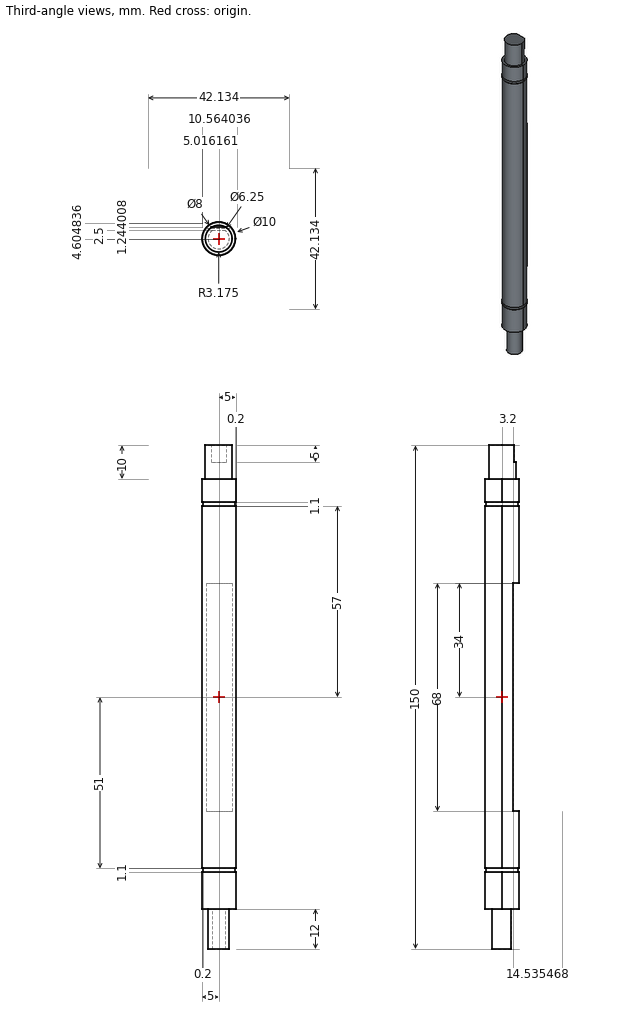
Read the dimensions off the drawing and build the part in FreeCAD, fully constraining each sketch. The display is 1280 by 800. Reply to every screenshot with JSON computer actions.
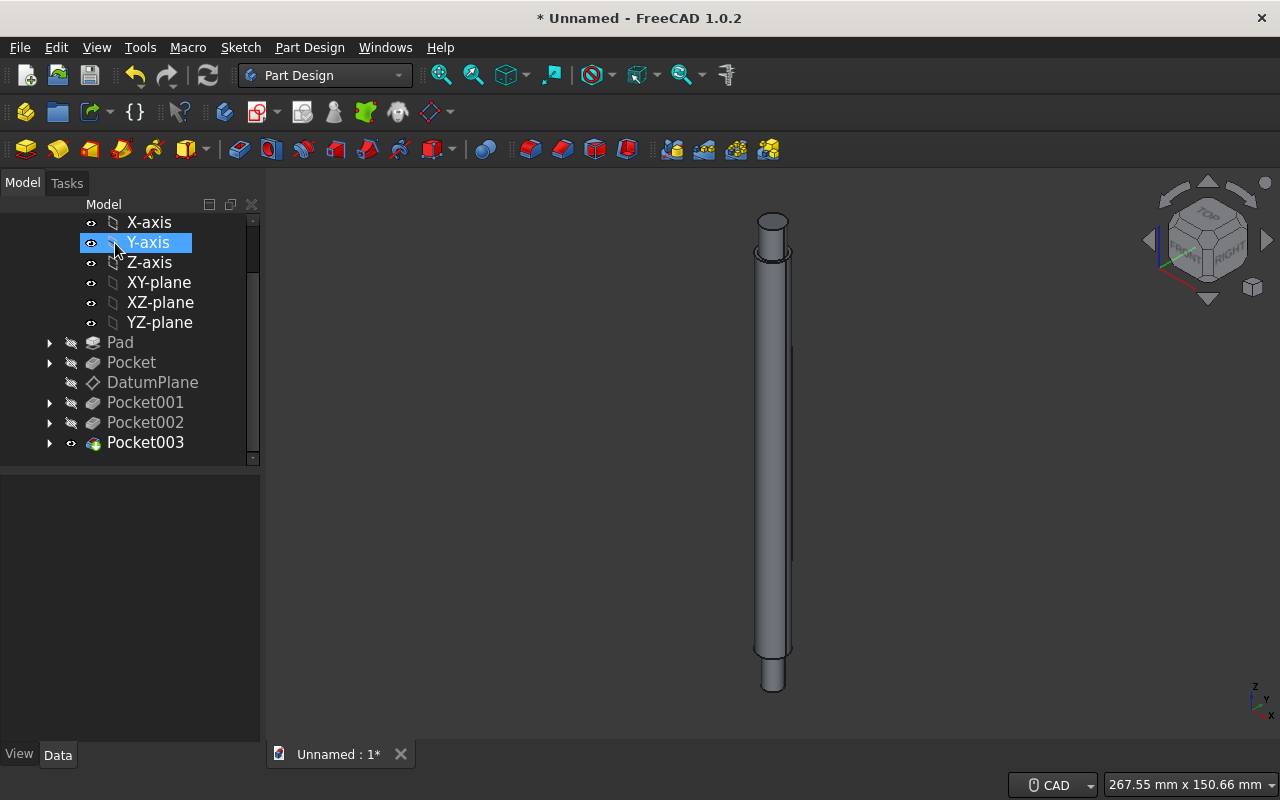
{"action": "left_click", "coordinate": [773, 220]}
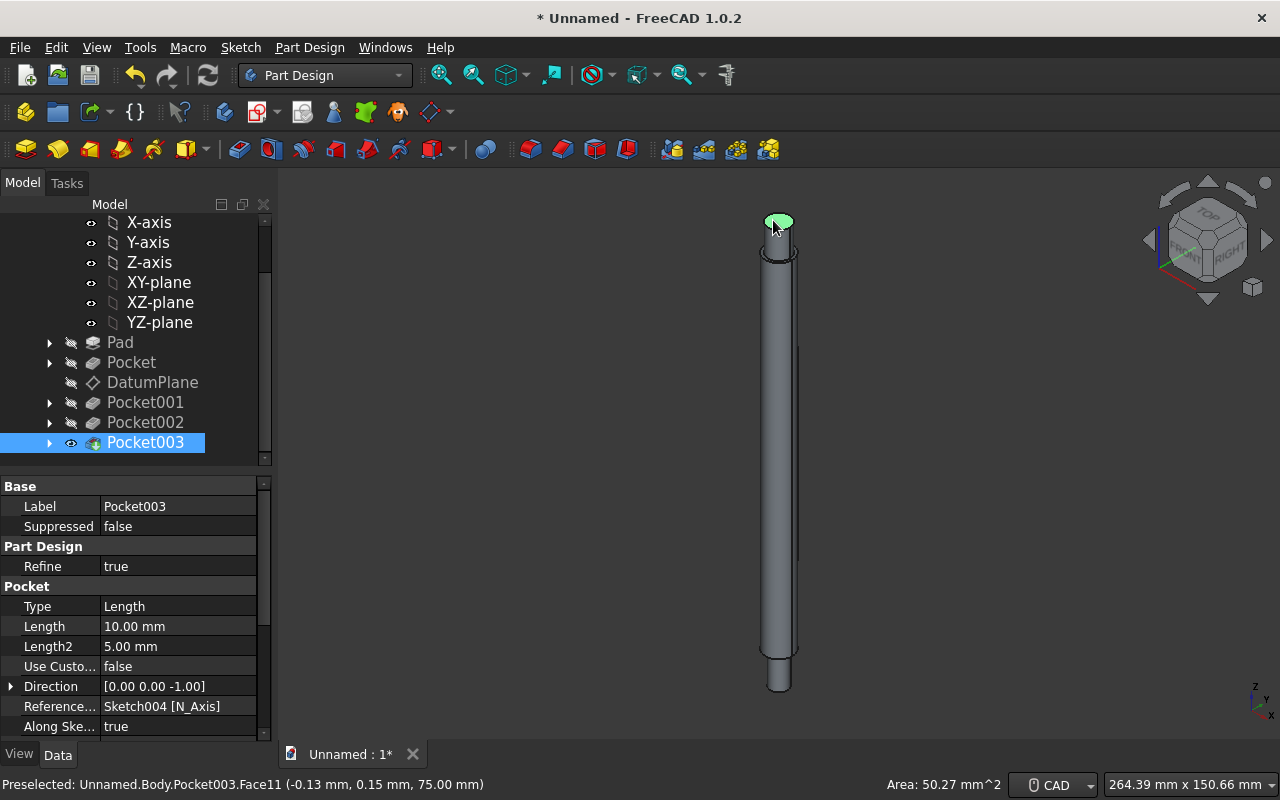
{"action": "left_click", "coordinate": [258, 112]}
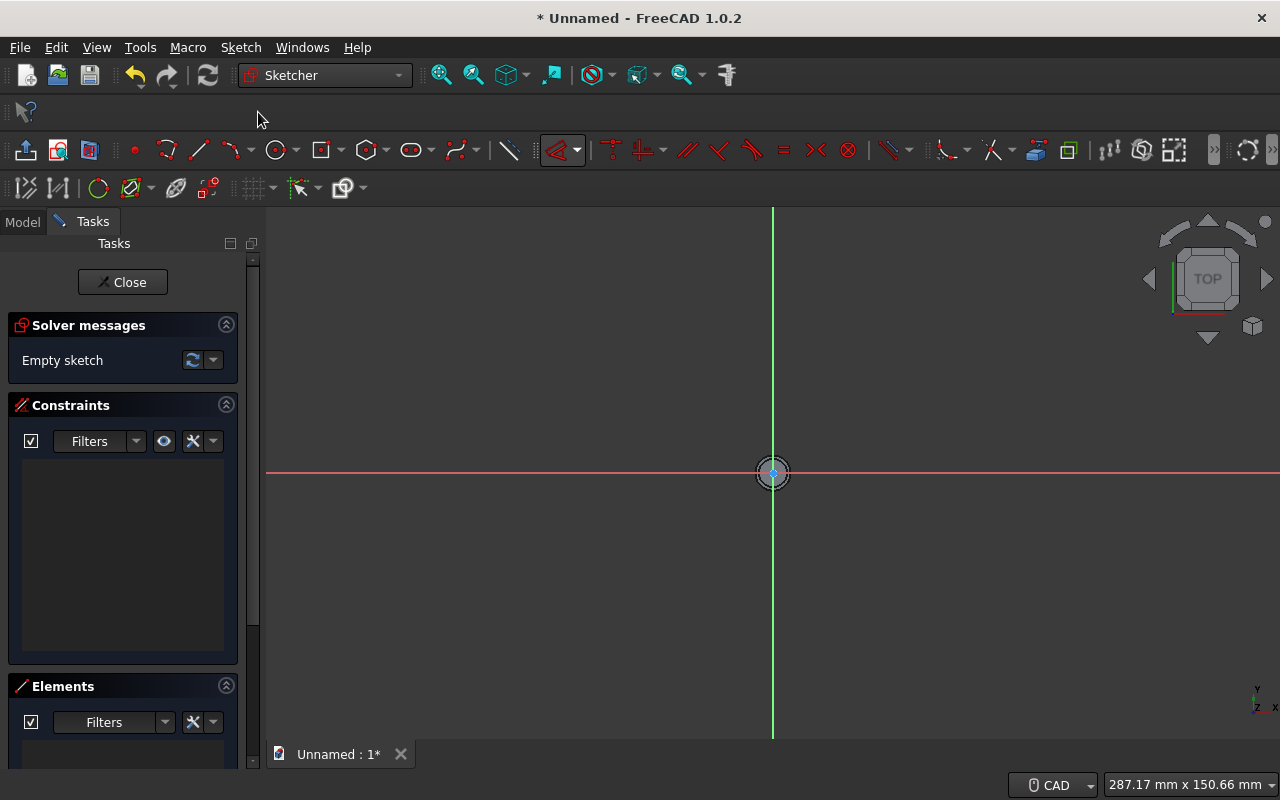
{"action": "scroll", "coordinate": [778, 464], "scroll_direction": "up", "scroll_amount": 14}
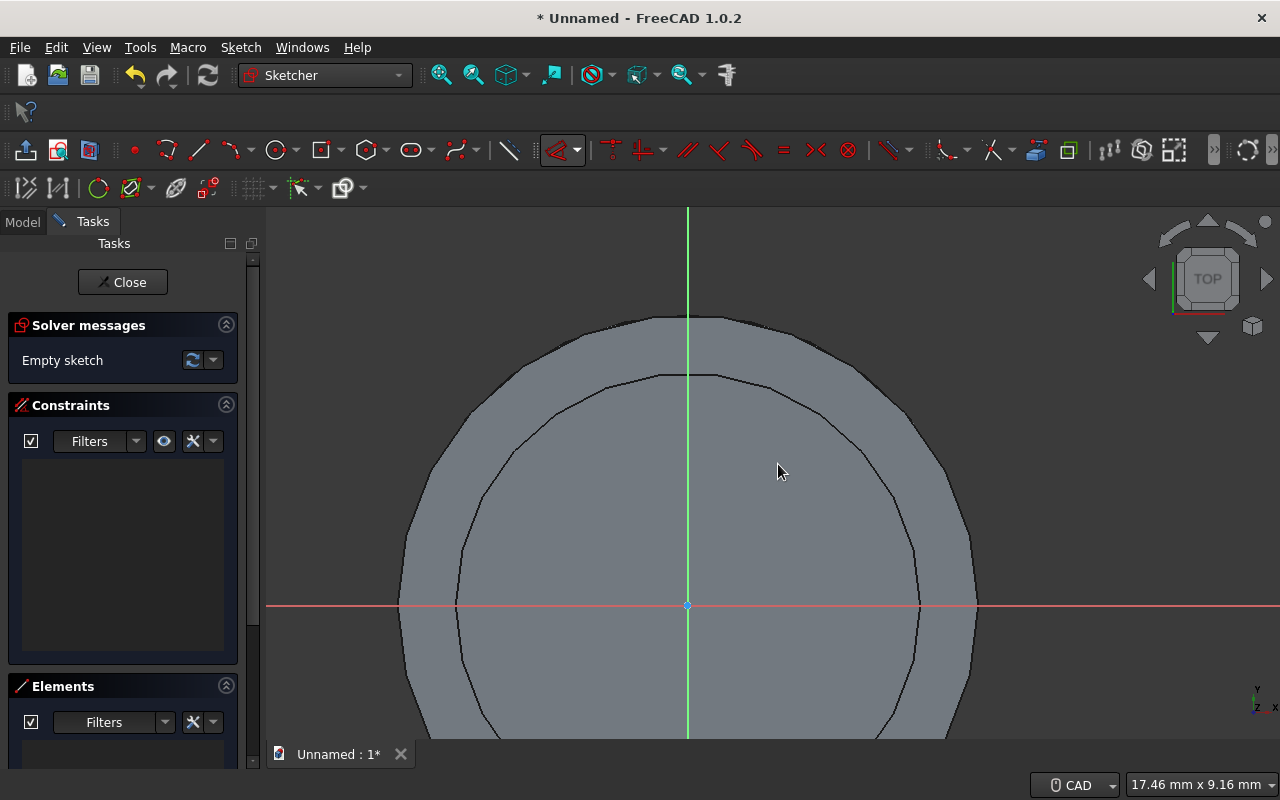
{"action": "key", "text": "g r"}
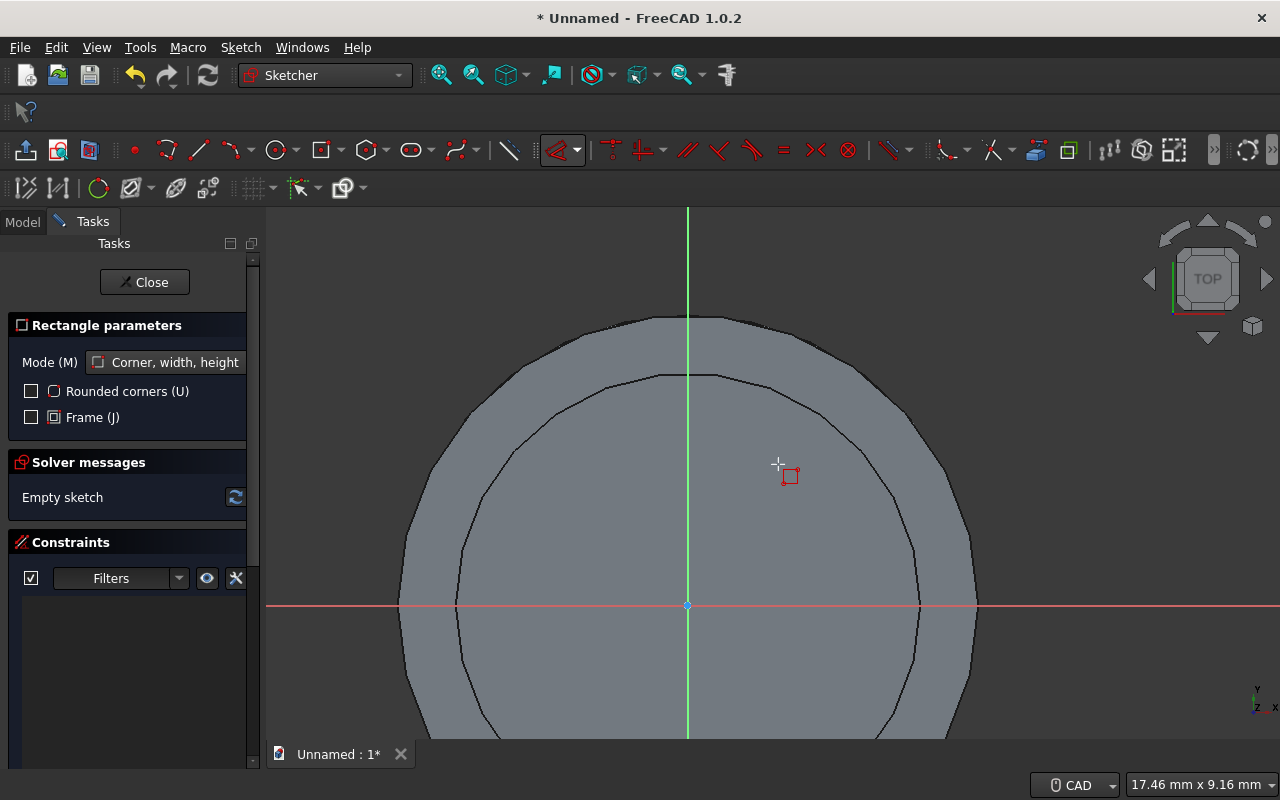
{"action": "left_click", "coordinate": [397, 338]}
{"action": "left_click", "coordinate": [1010, 410]}
{"action": "key", "text": "Escape"}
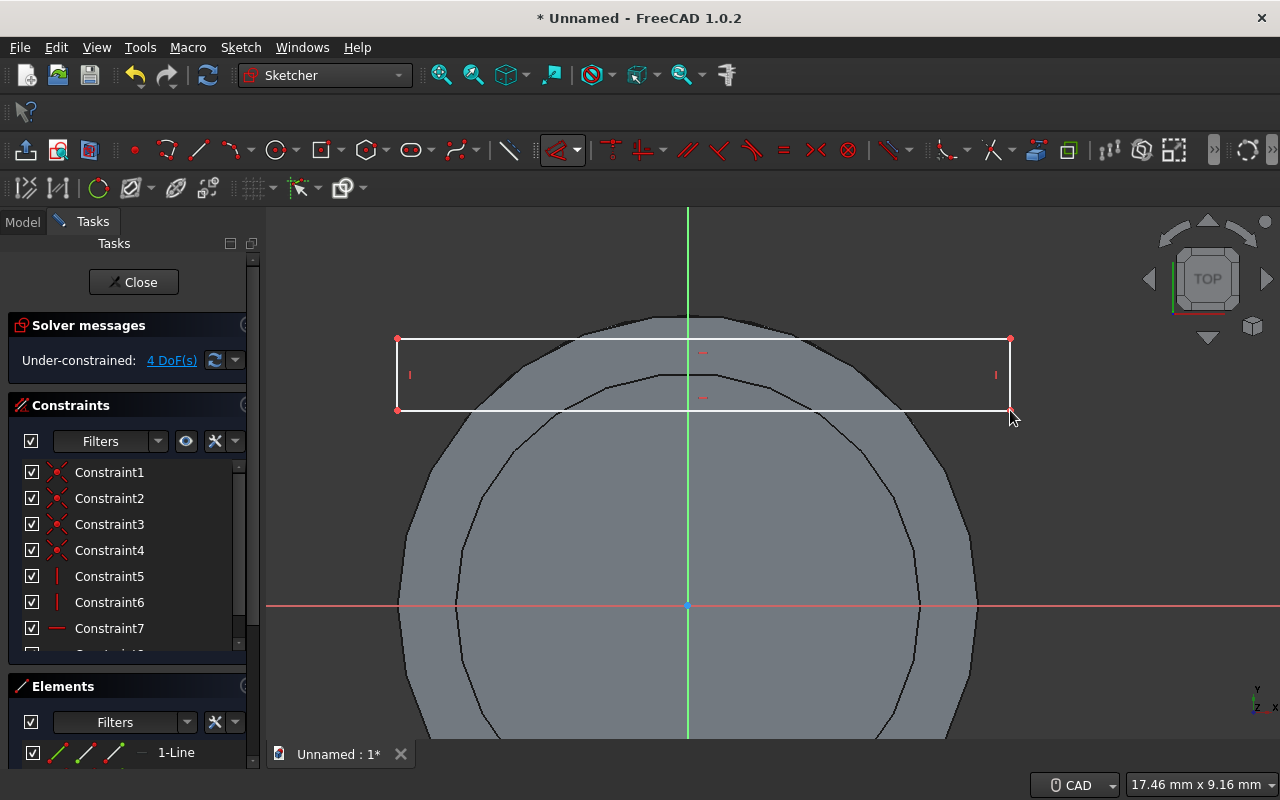
{"action": "left_click", "coordinate": [397, 361]}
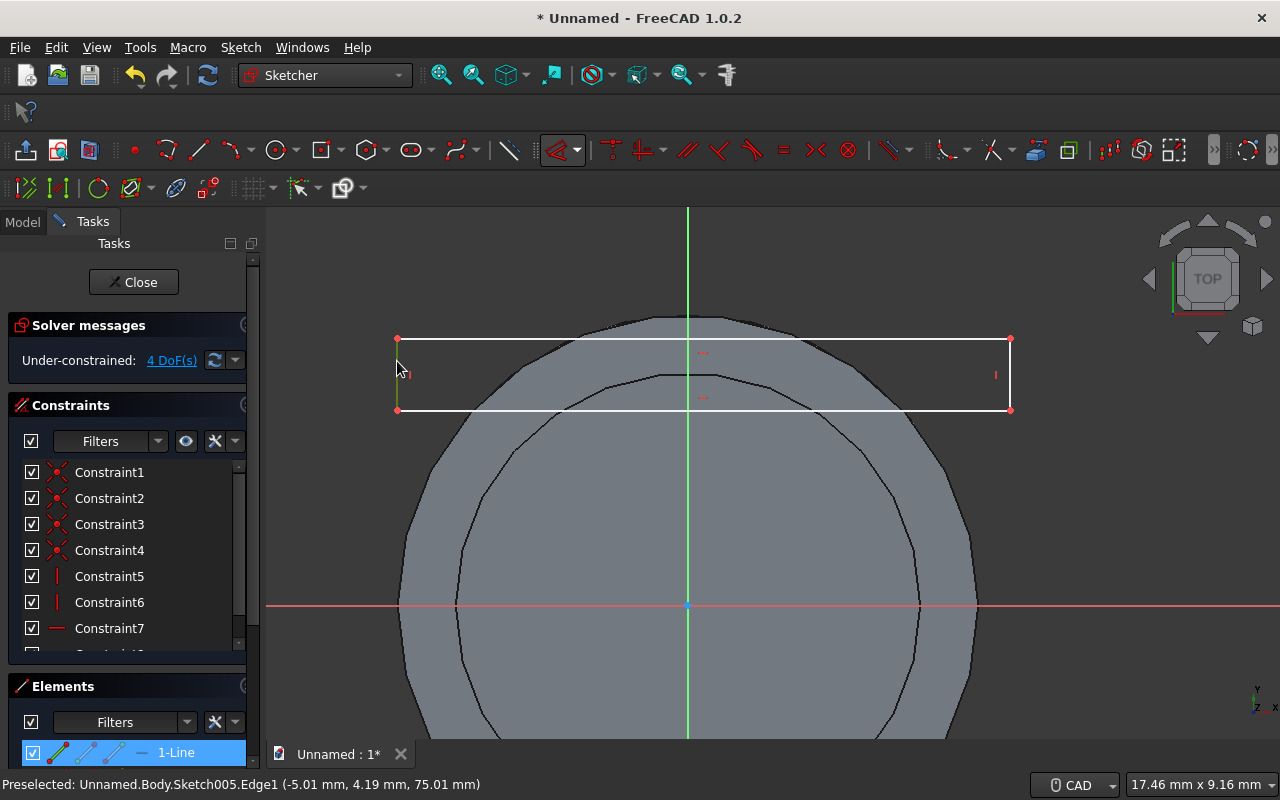
{"action": "left_click", "coordinate": [580, 150]}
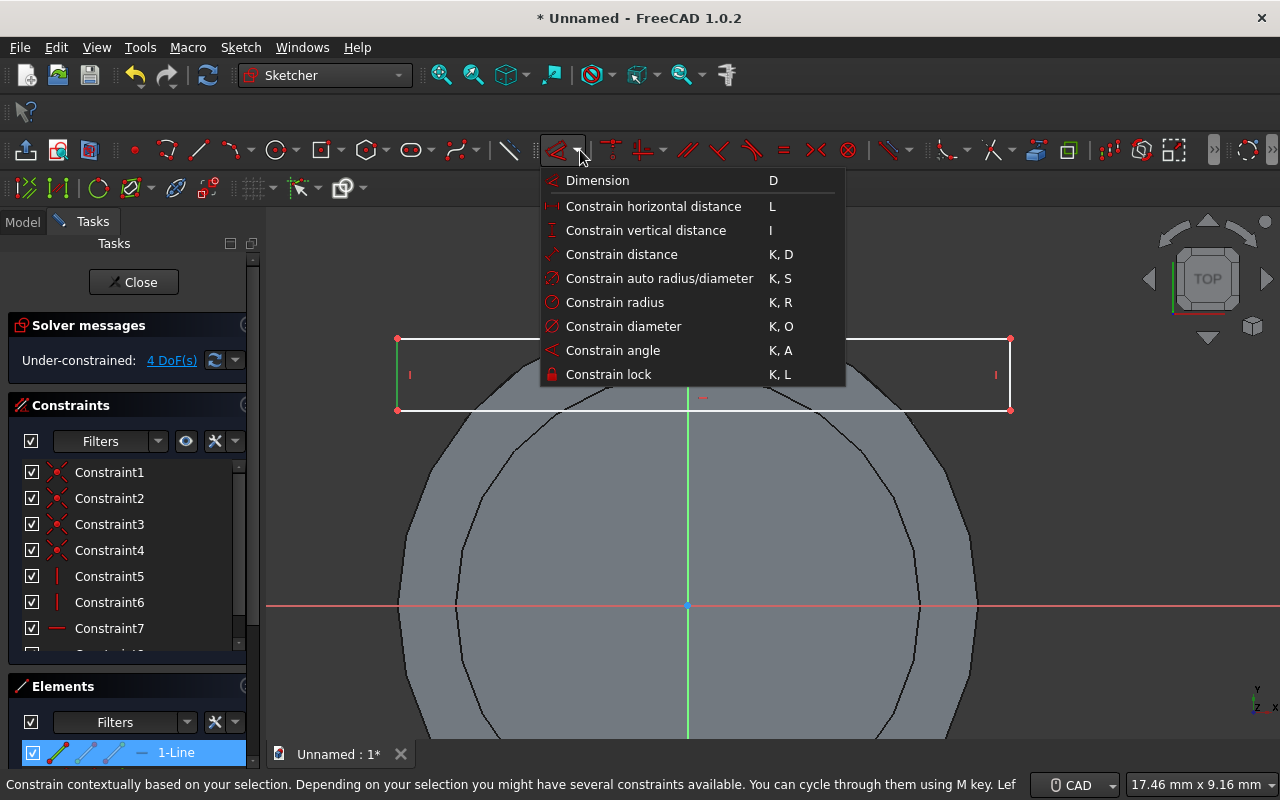
{"action": "left_click", "coordinate": [693, 230]}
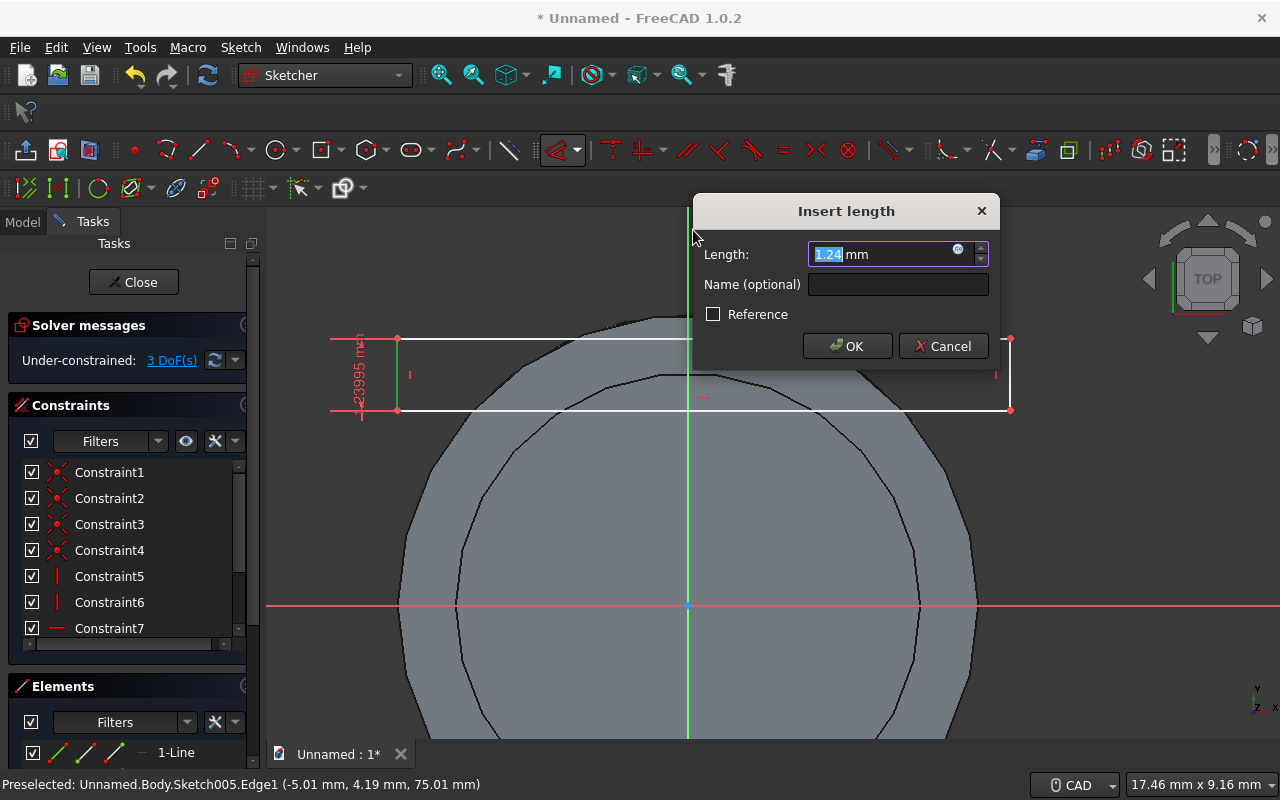
{"action": "type", "text": "1.244008"}
{"action": "key", "text": "Return"}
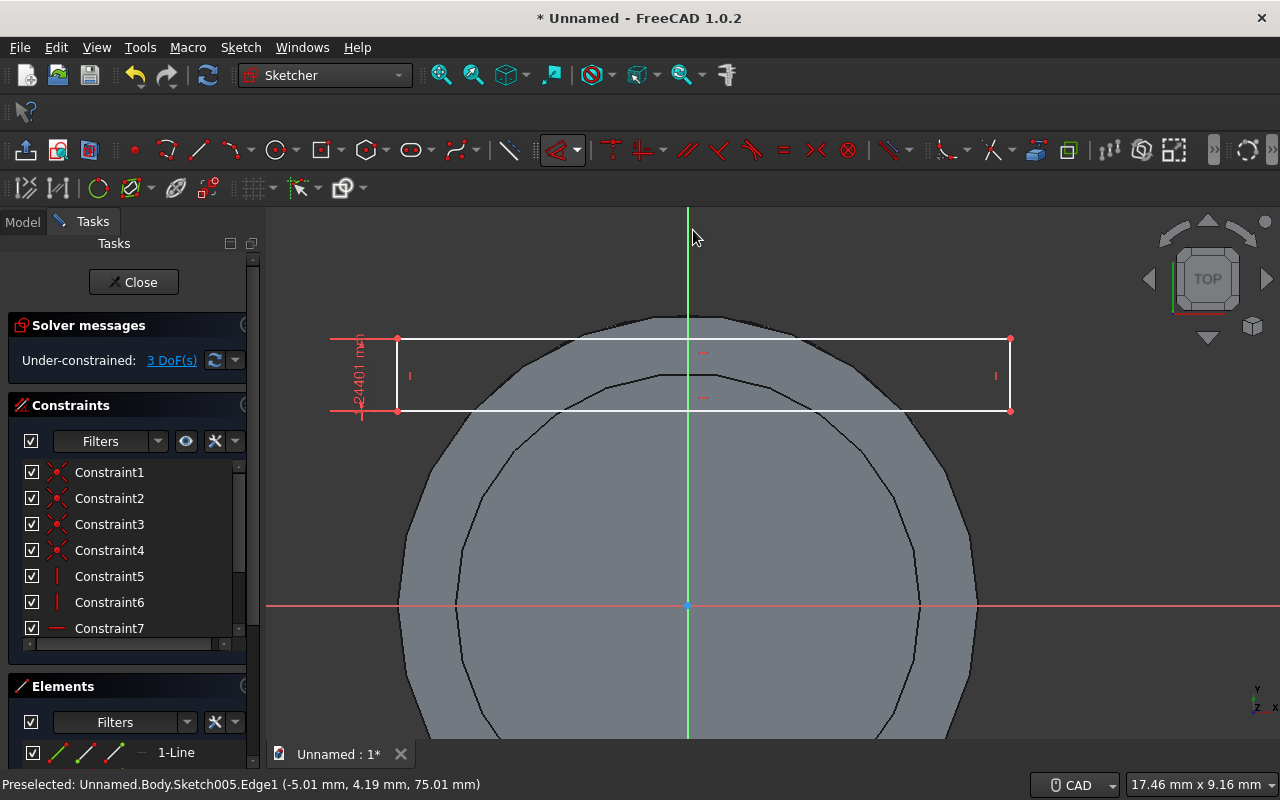
{"action": "left_click", "coordinate": [581, 411]}